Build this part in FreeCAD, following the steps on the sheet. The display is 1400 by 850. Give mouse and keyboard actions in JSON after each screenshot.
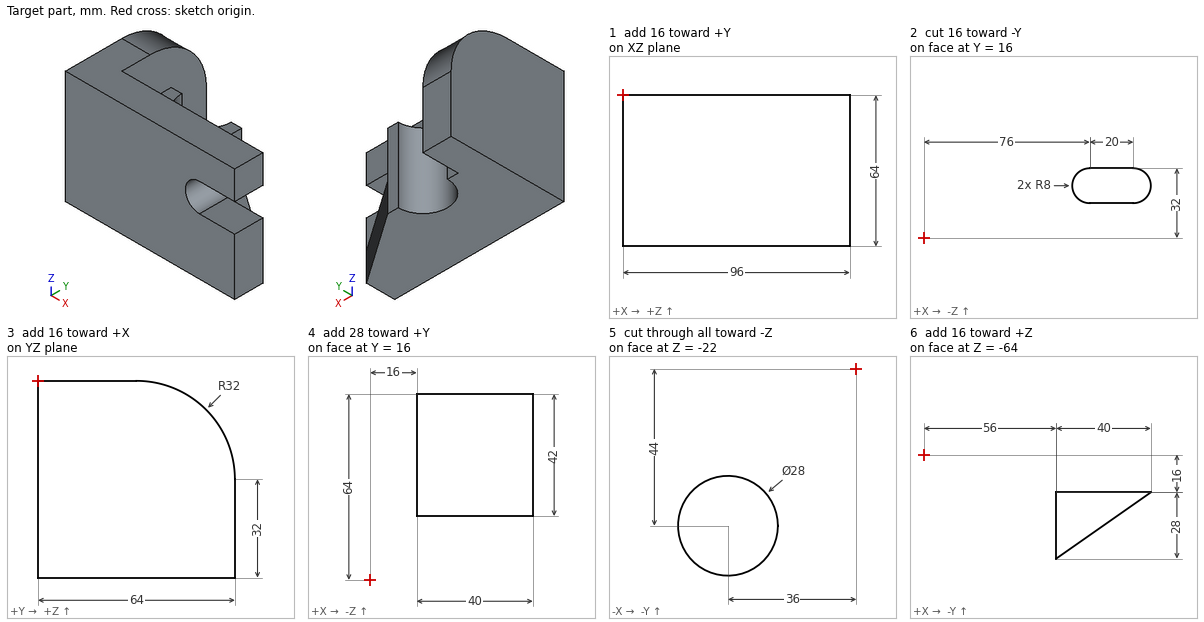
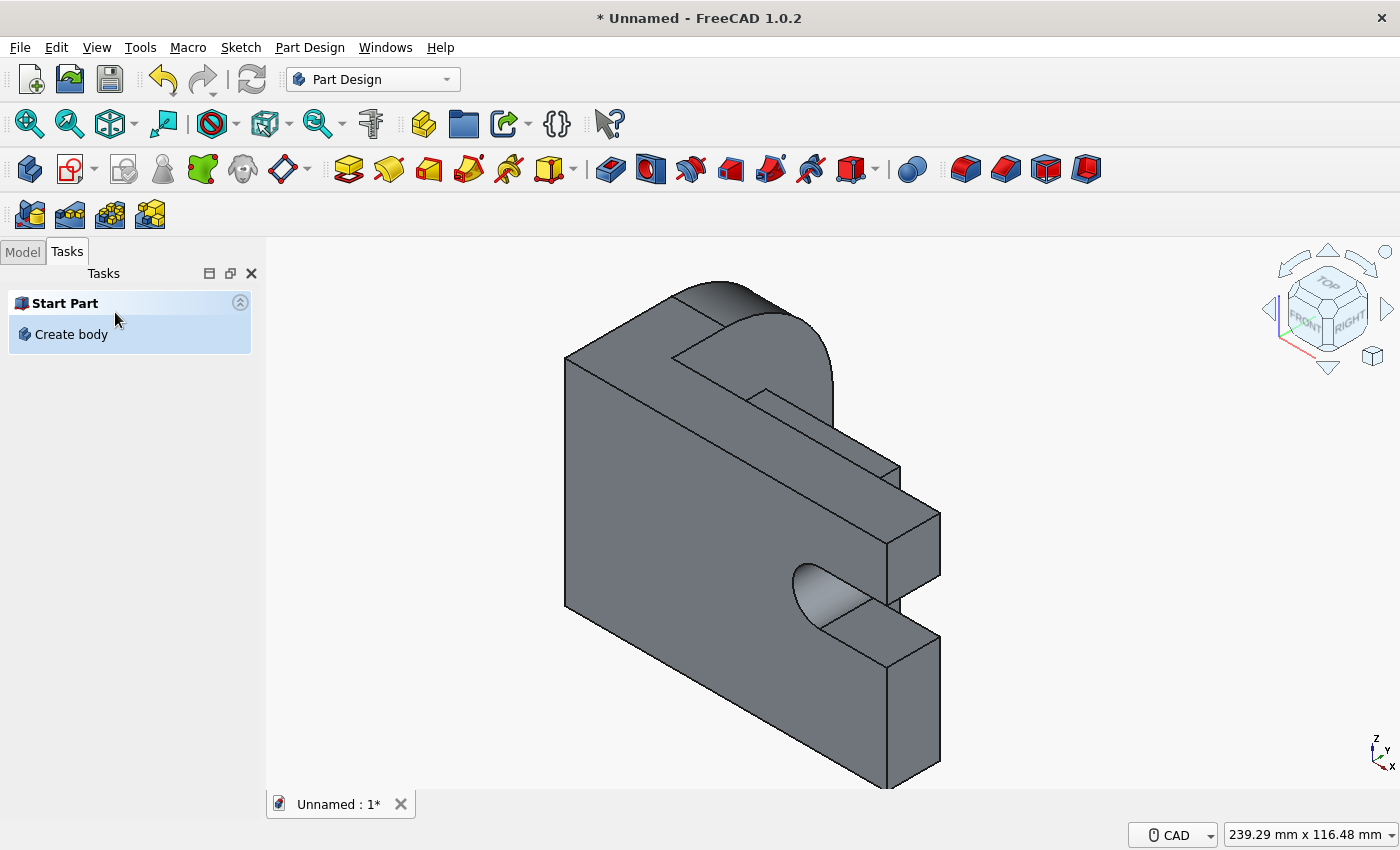
{"action": "key", "text": "v f"}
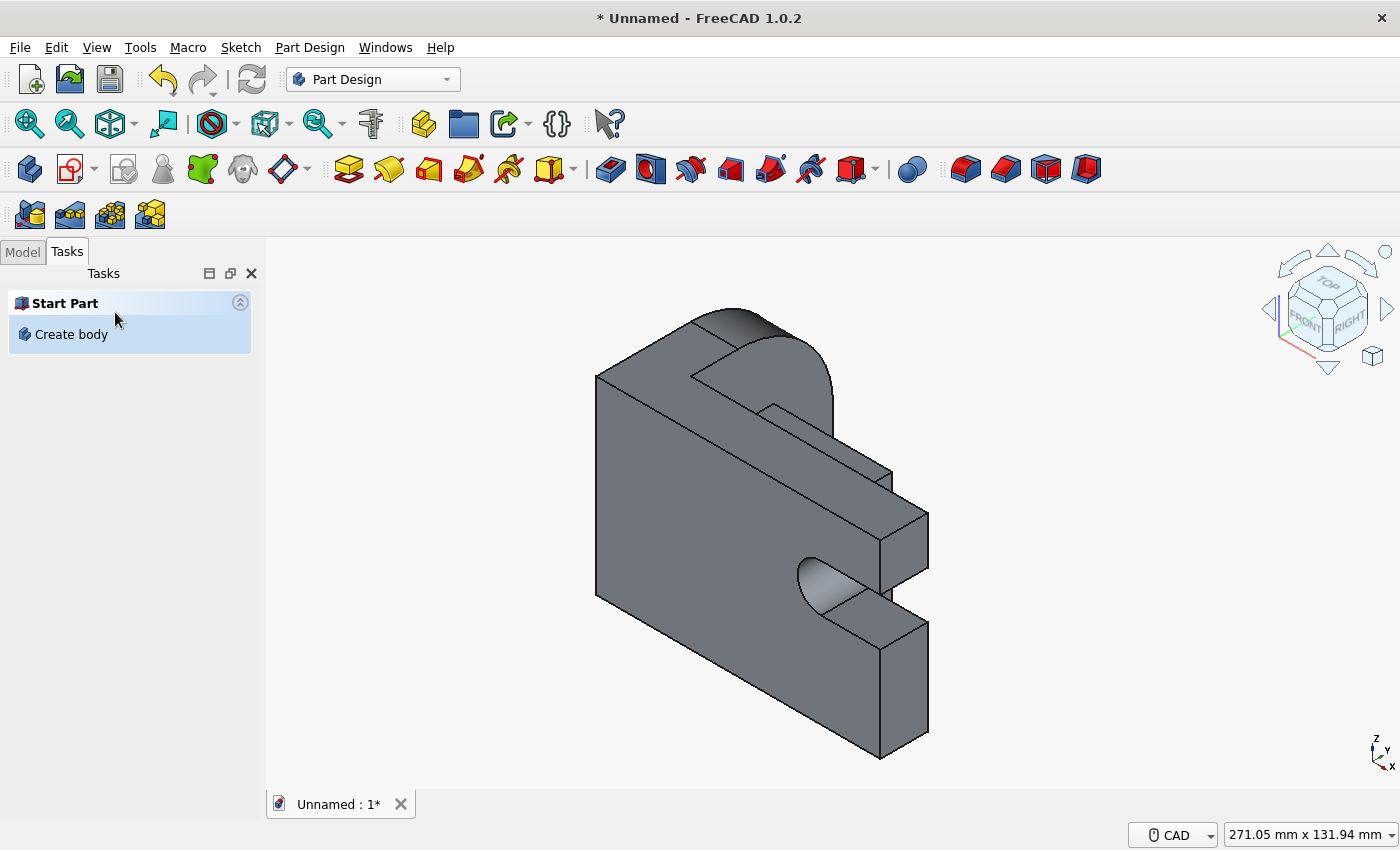
{"action": "key", "text": "2"}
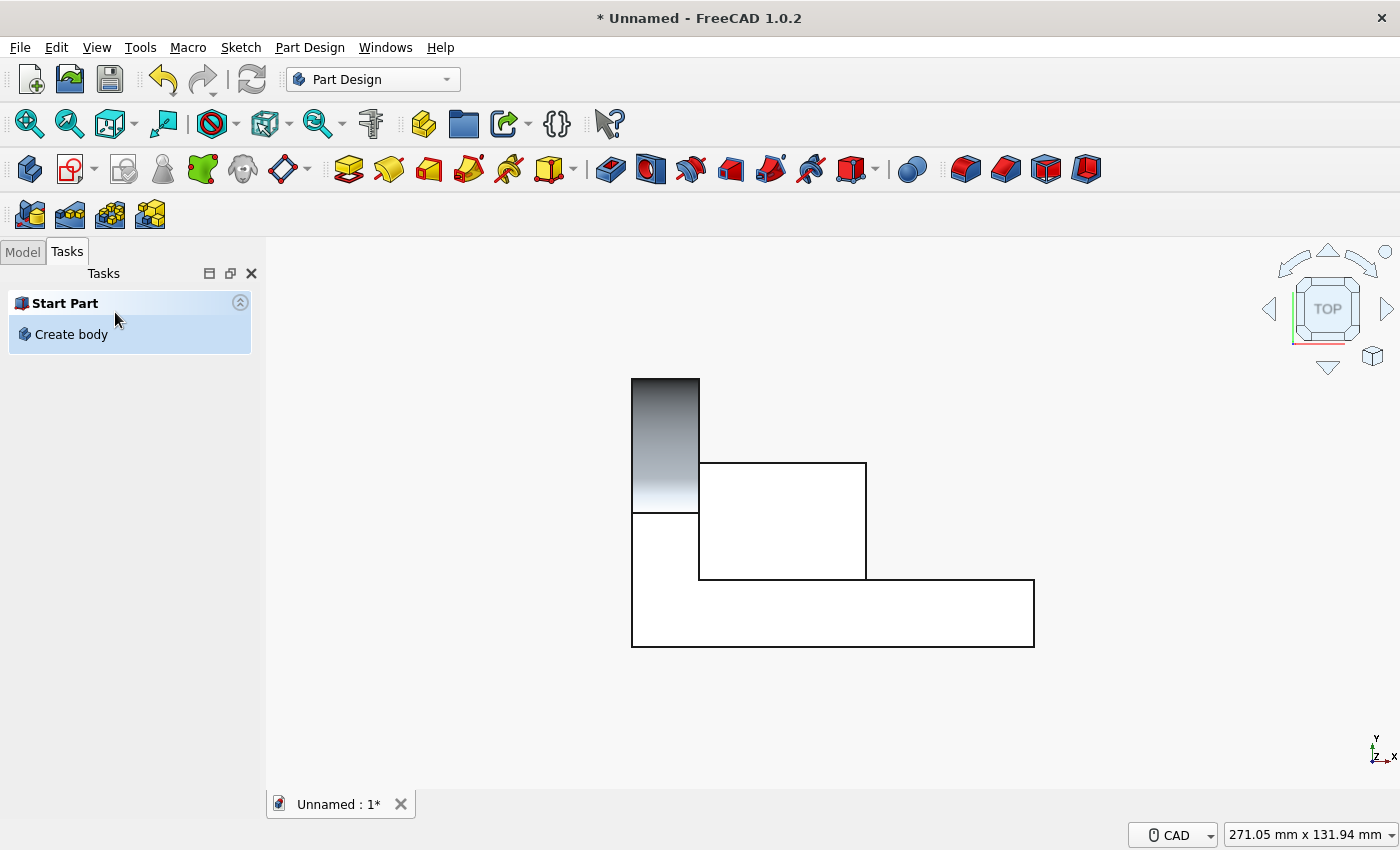
{"action": "left_click", "coordinate": [807, 520]}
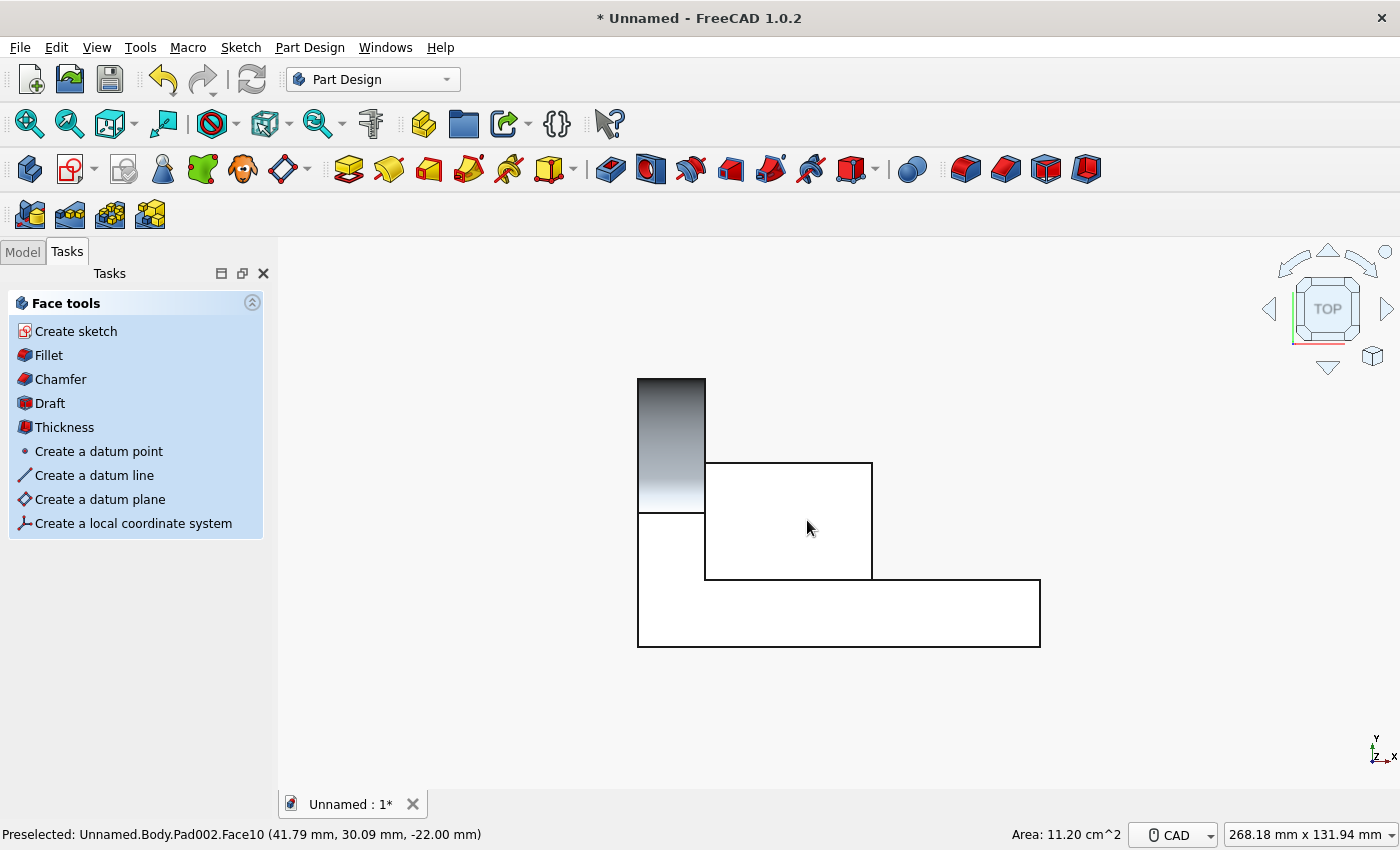
{"action": "left_click", "coordinate": [70, 170]}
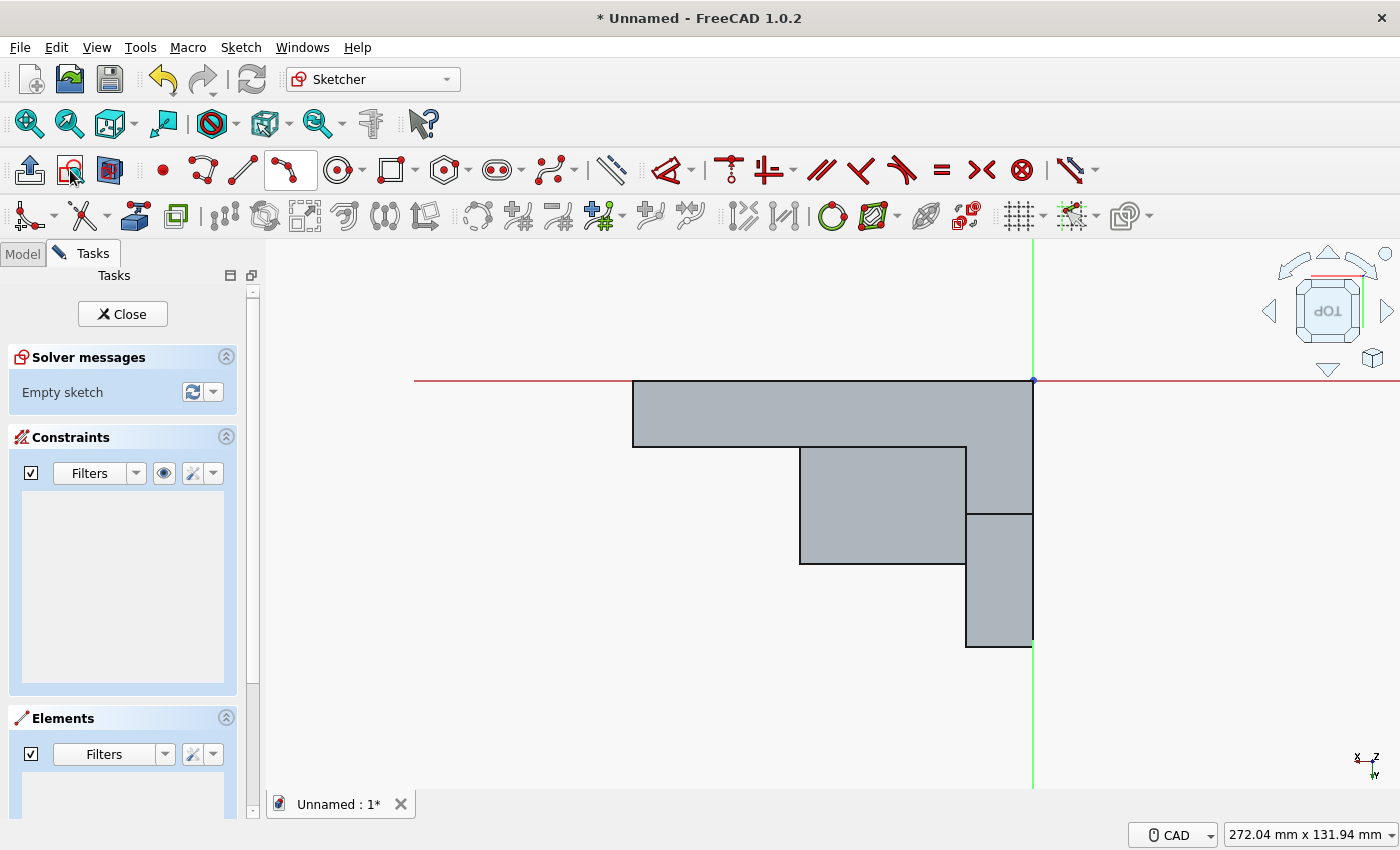
{"action": "left_click", "coordinate": [110, 170]}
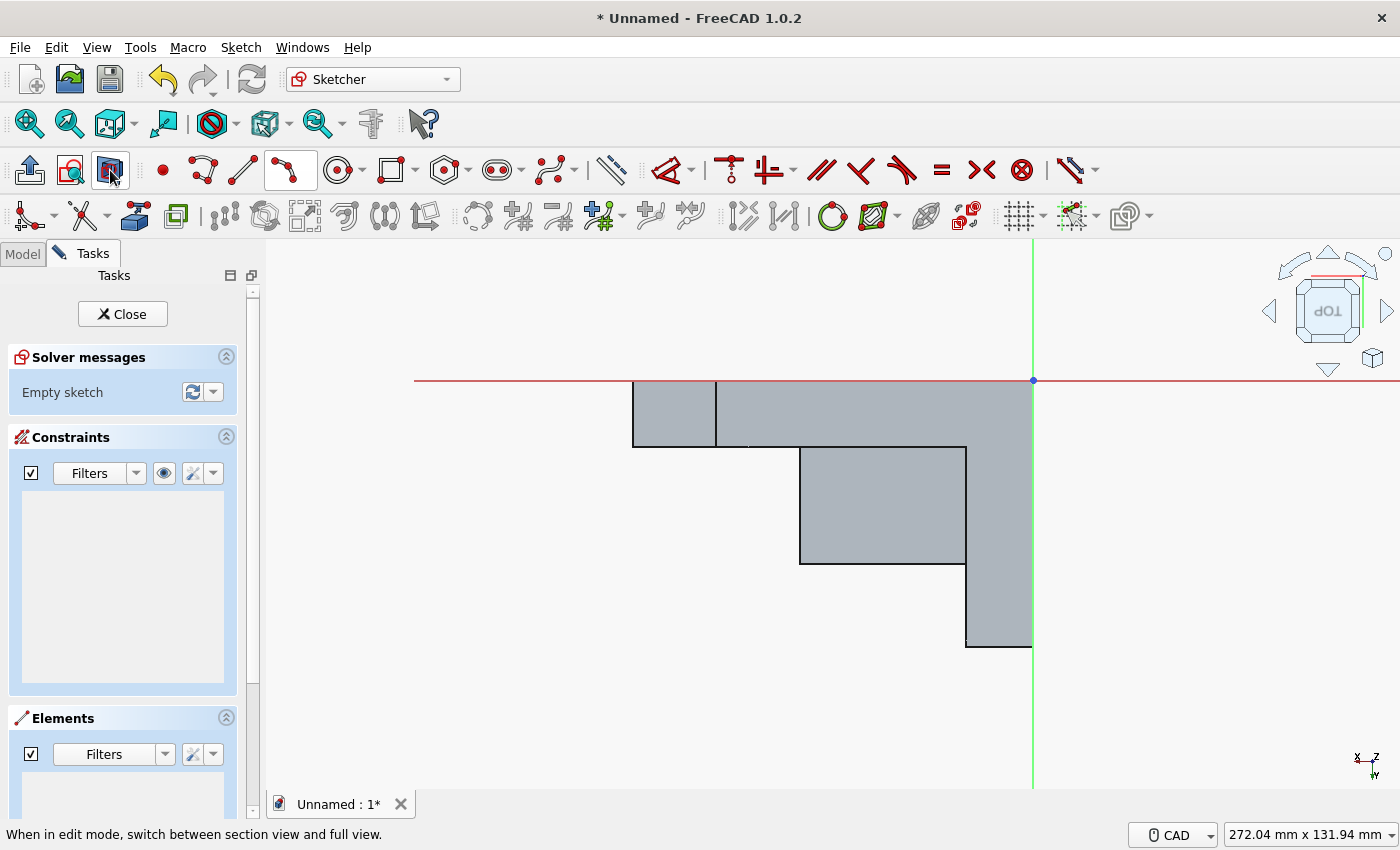
{"action": "scroll", "coordinate": [1235, 476], "scroll_direction": "up", "scroll_amount": 2}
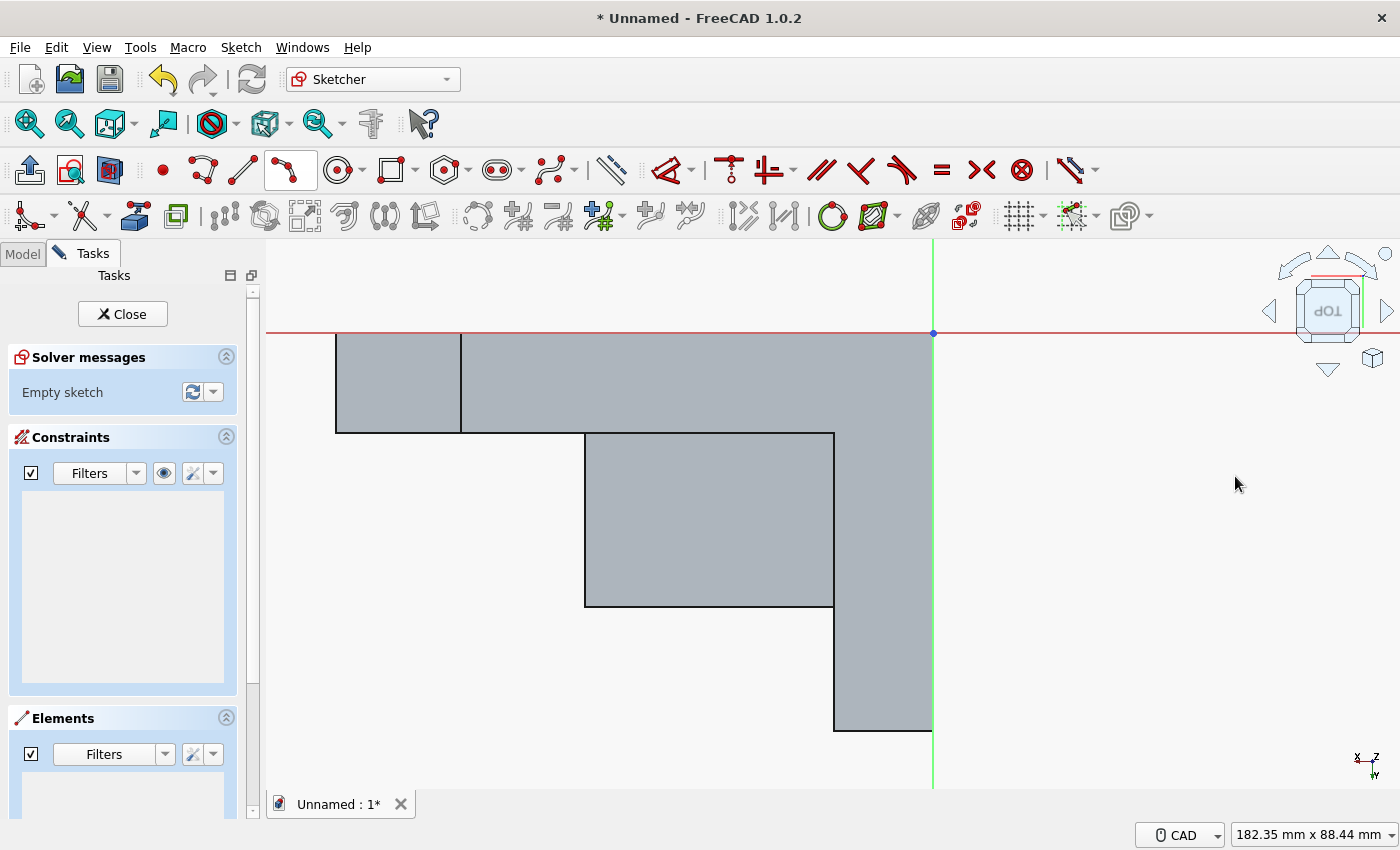
{"action": "left_click", "coordinate": [338, 170]}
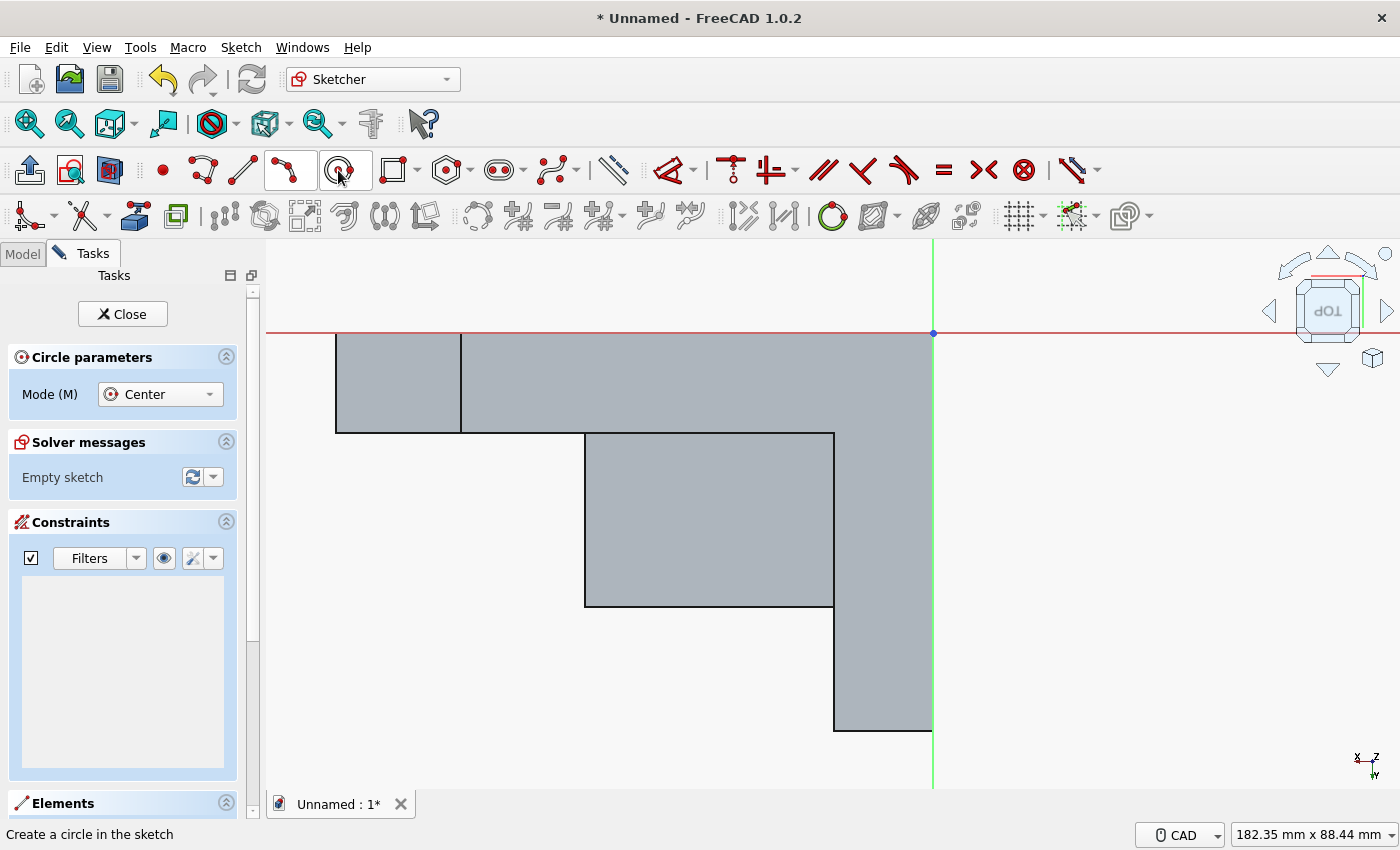
{"action": "left_click", "coordinate": [709, 607]}
{"action": "mouse_move", "coordinate": [771, 546]}